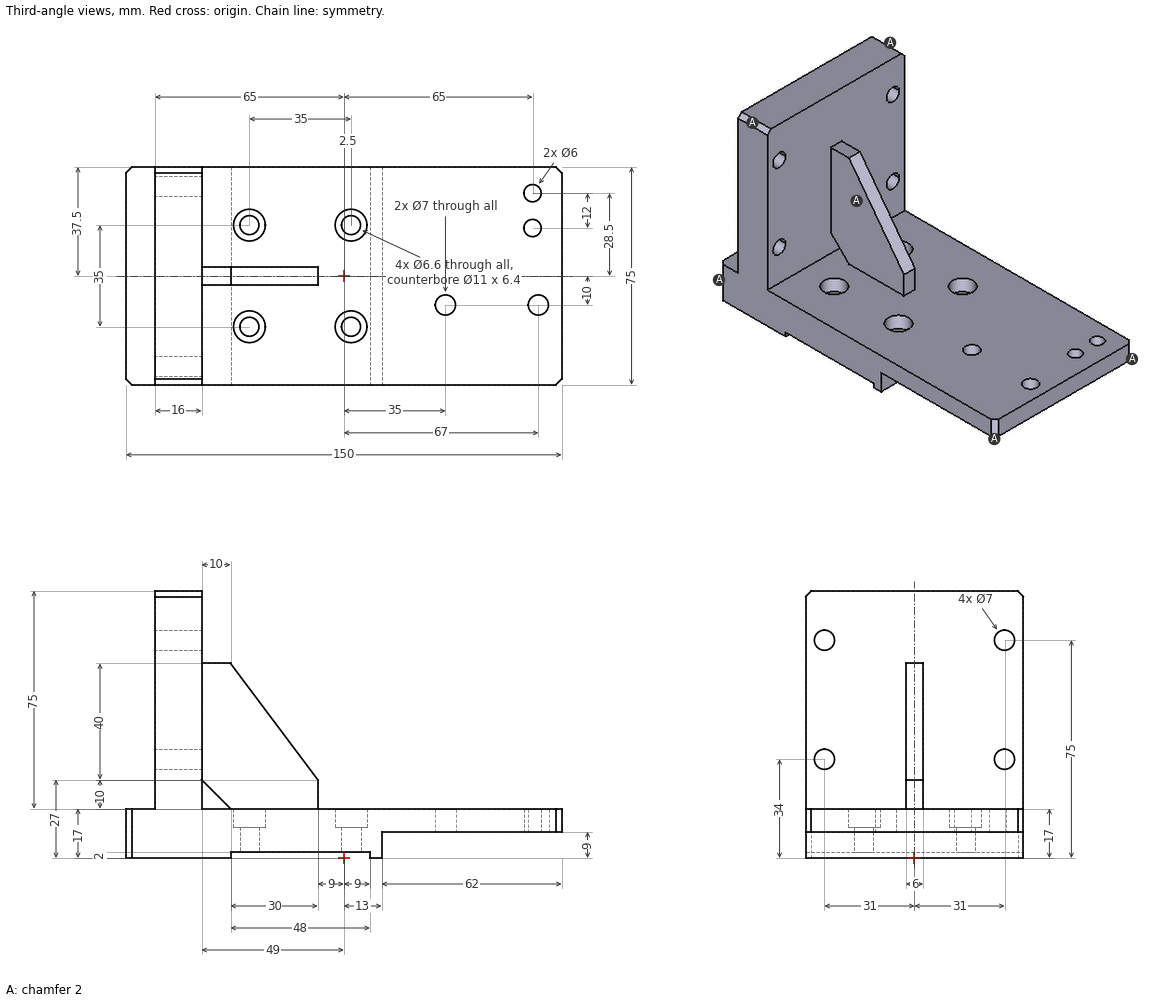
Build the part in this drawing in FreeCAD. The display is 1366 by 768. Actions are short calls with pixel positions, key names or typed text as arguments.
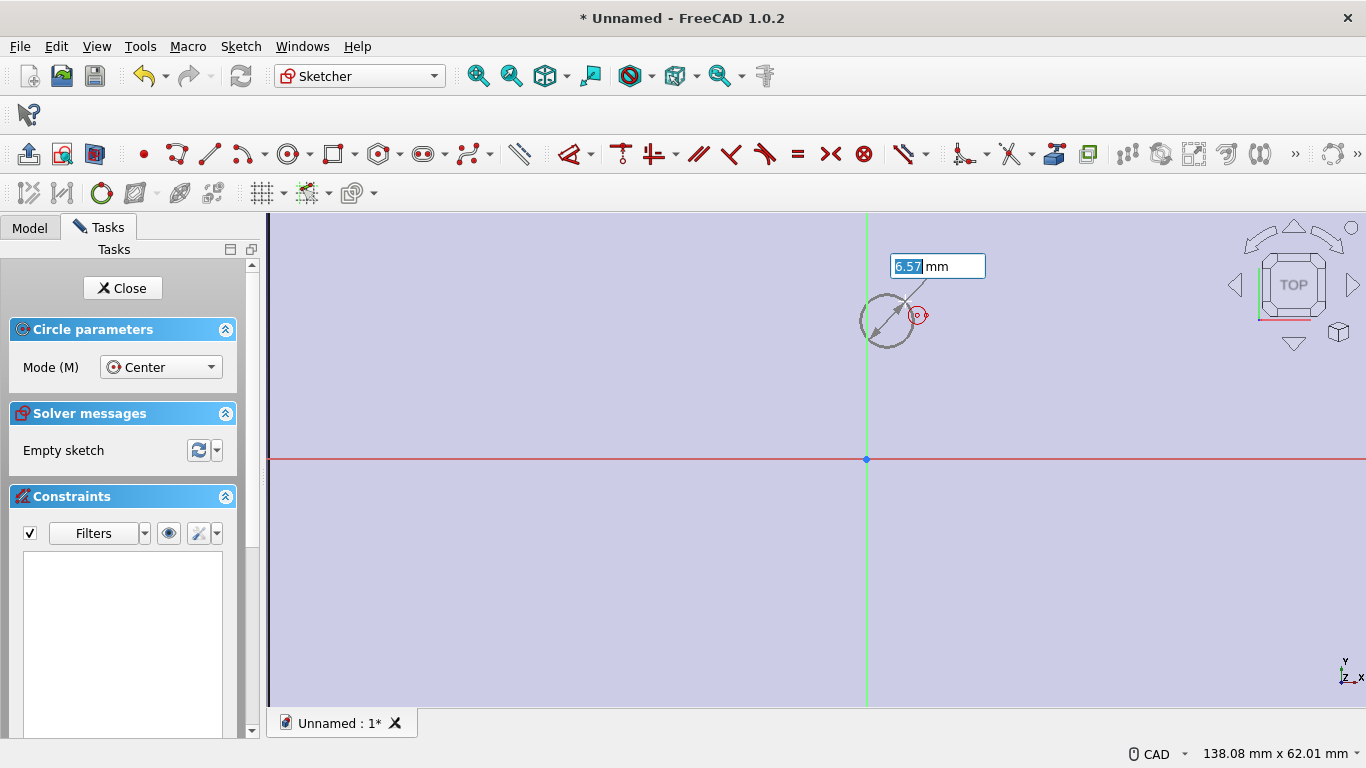
text(6.6)
key(Return)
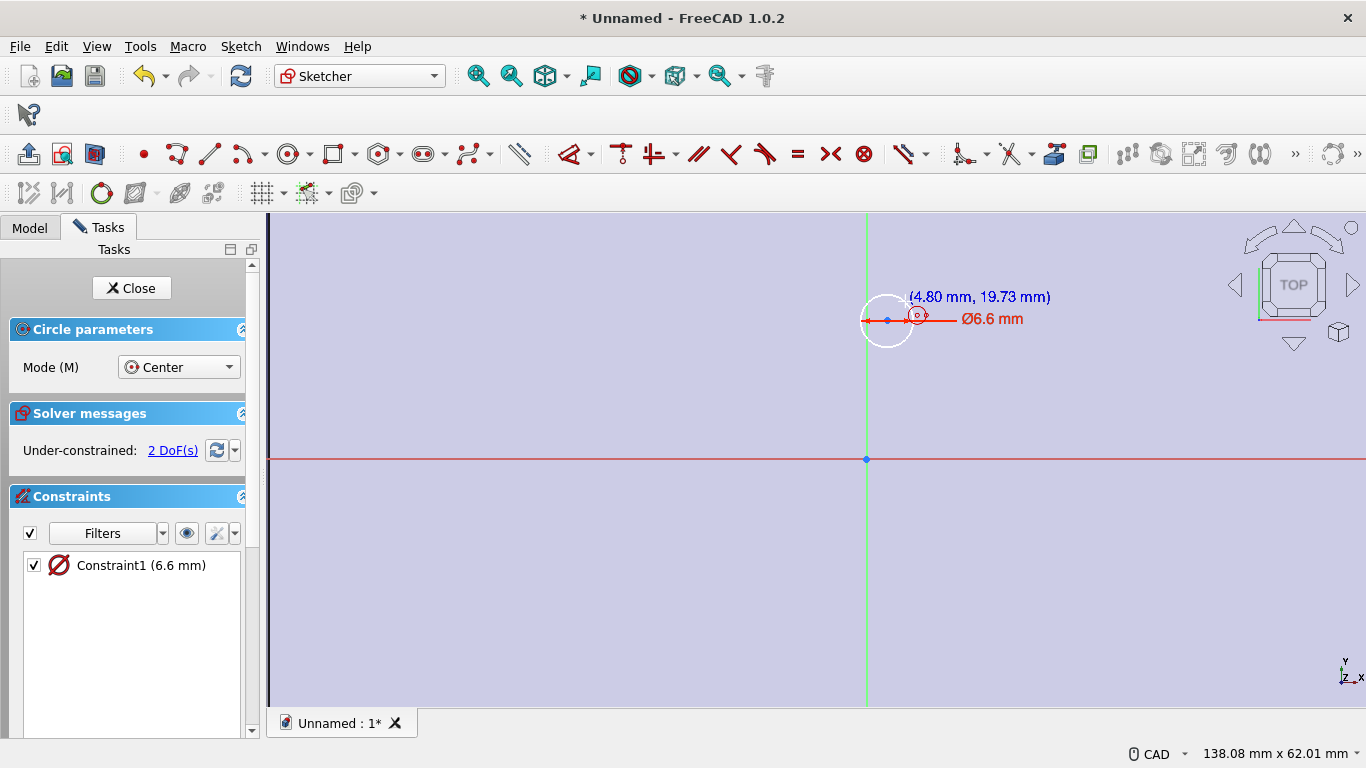
click(608, 320)
move(626, 301)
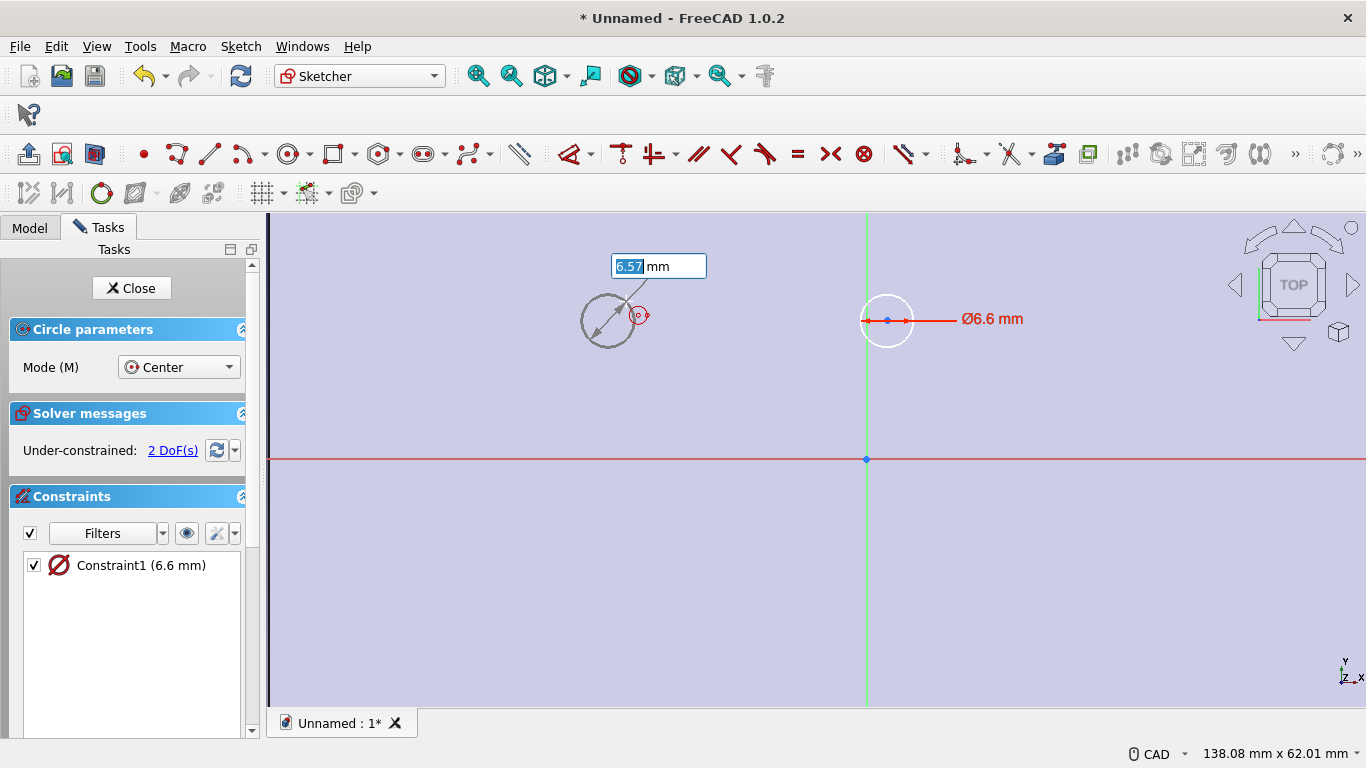
text(6.6)
key(Return)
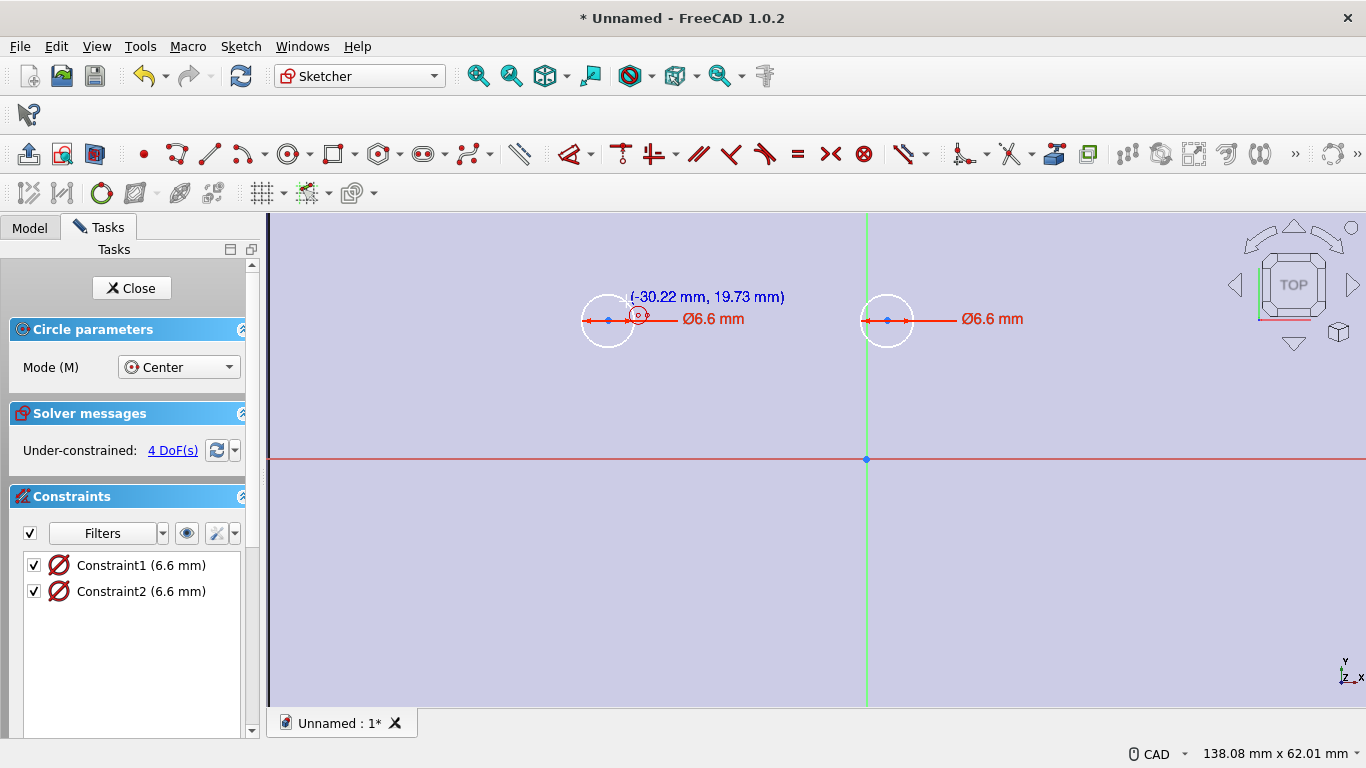
click(608, 599)
move(626, 580)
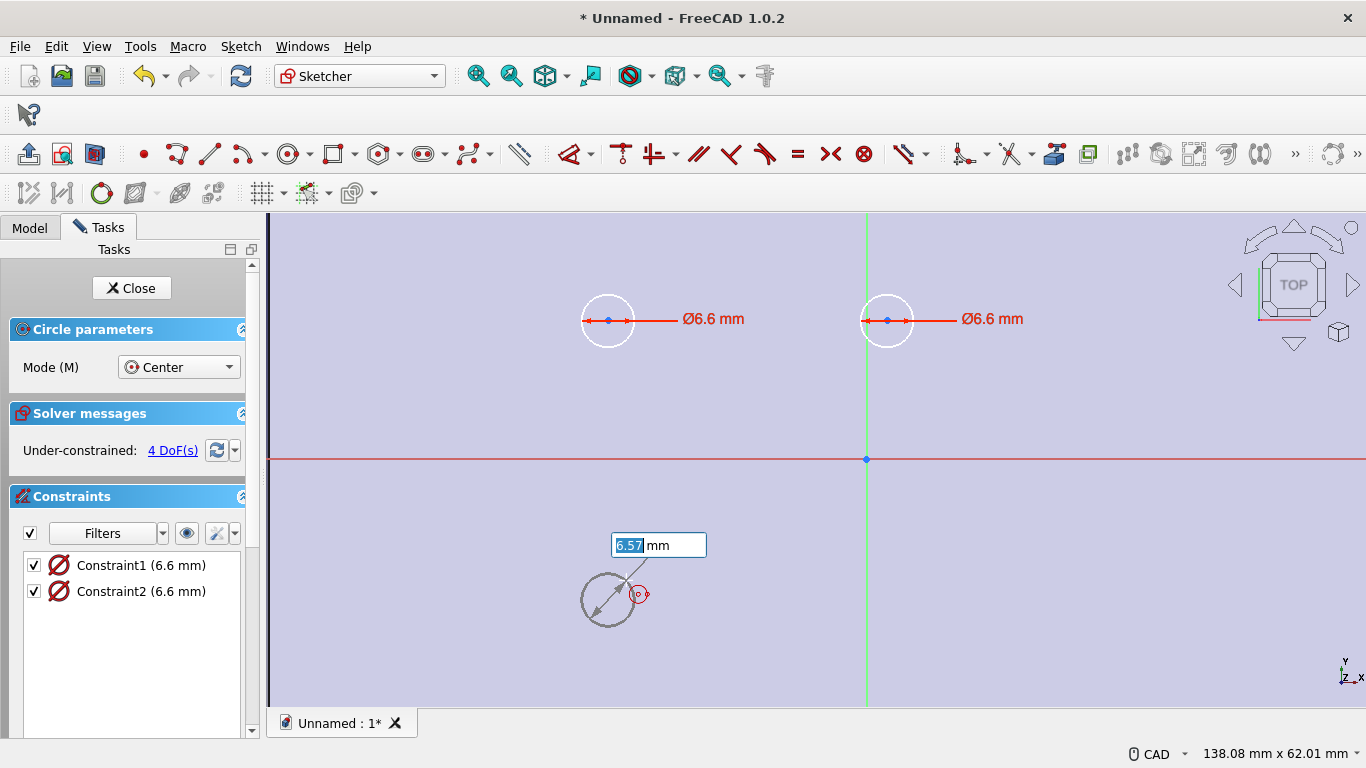
text(6.6)
key(Return)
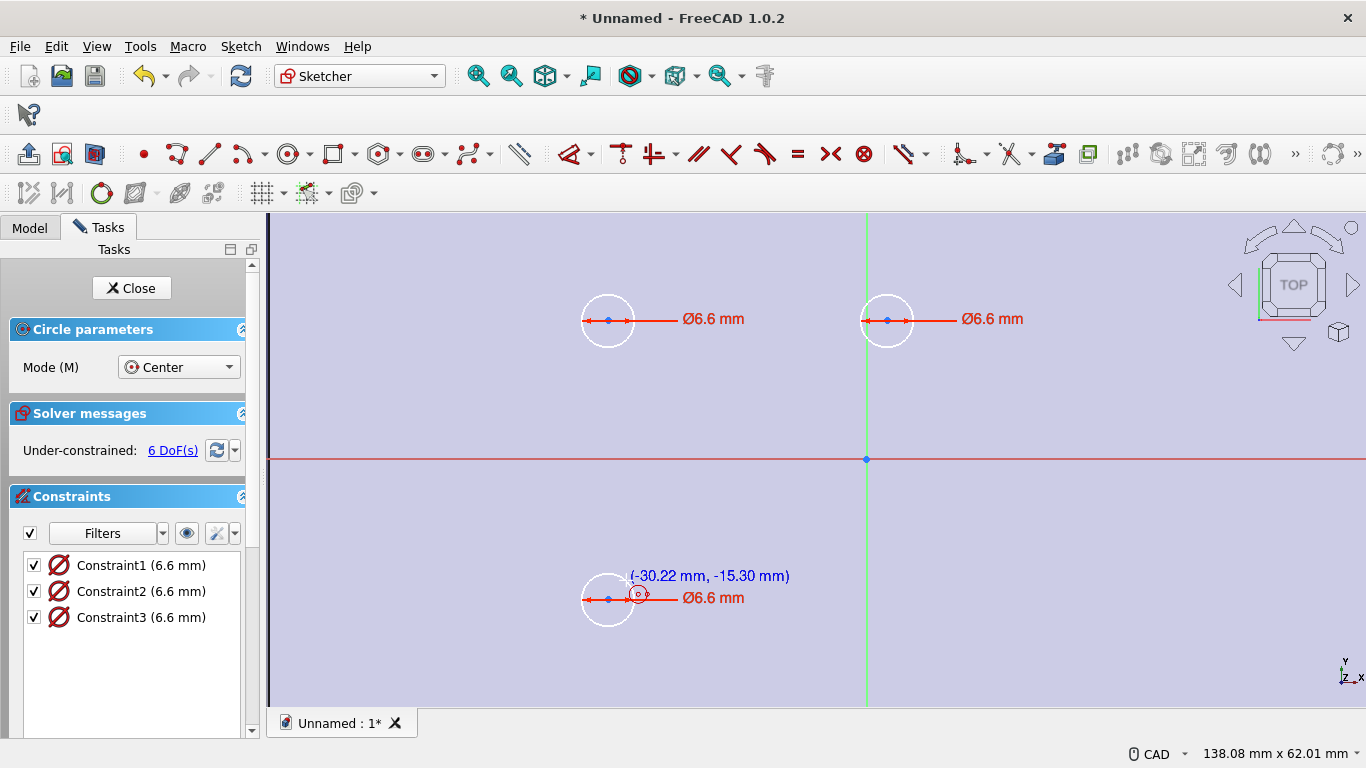
click(887, 599)
move(905, 580)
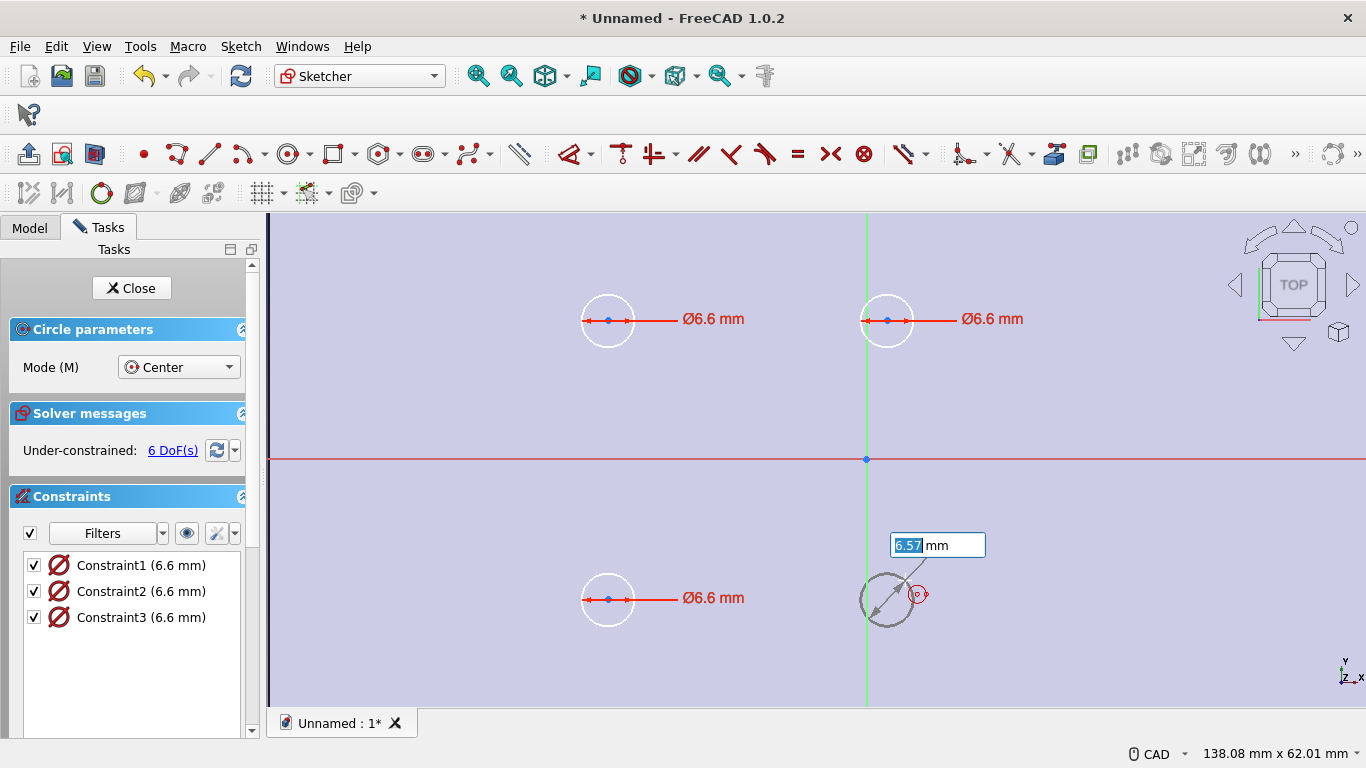
text(6.6)
key(Return)
key(Escape)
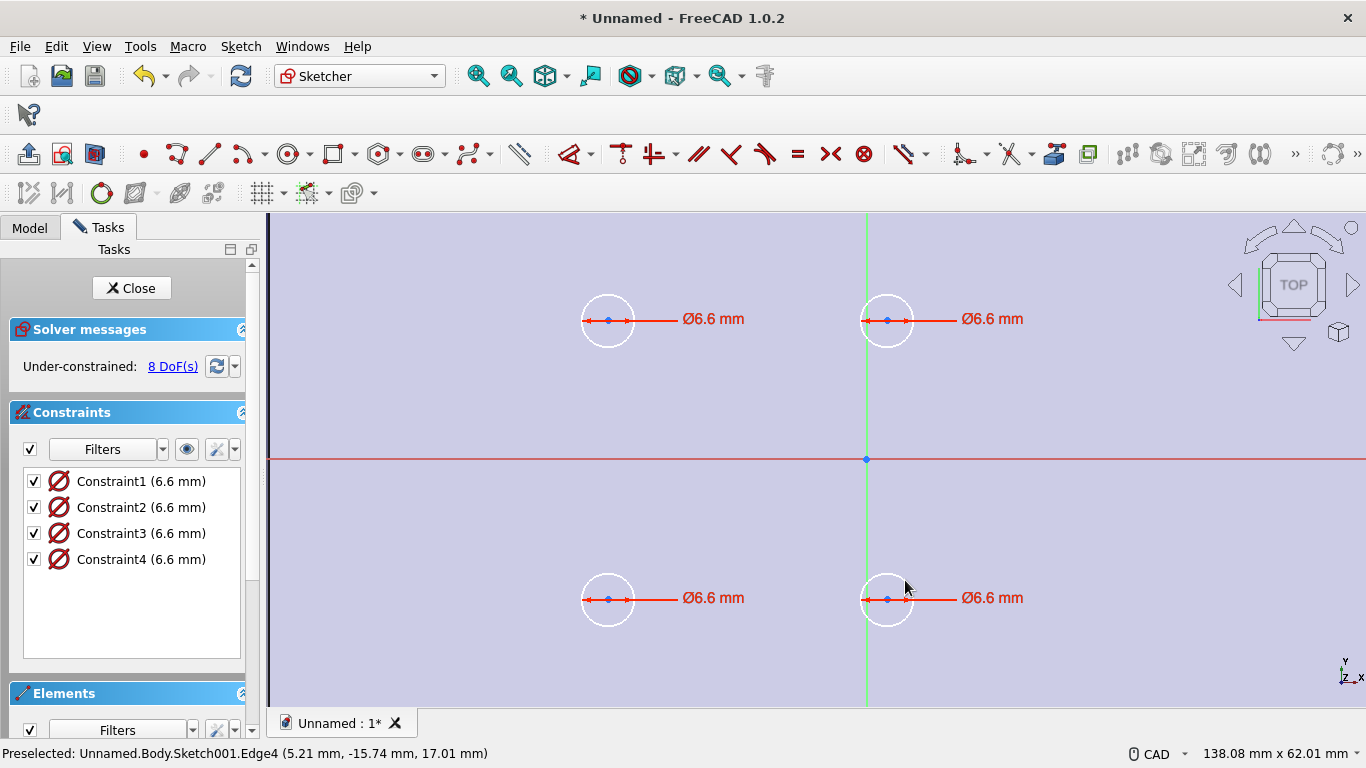
click(608, 321)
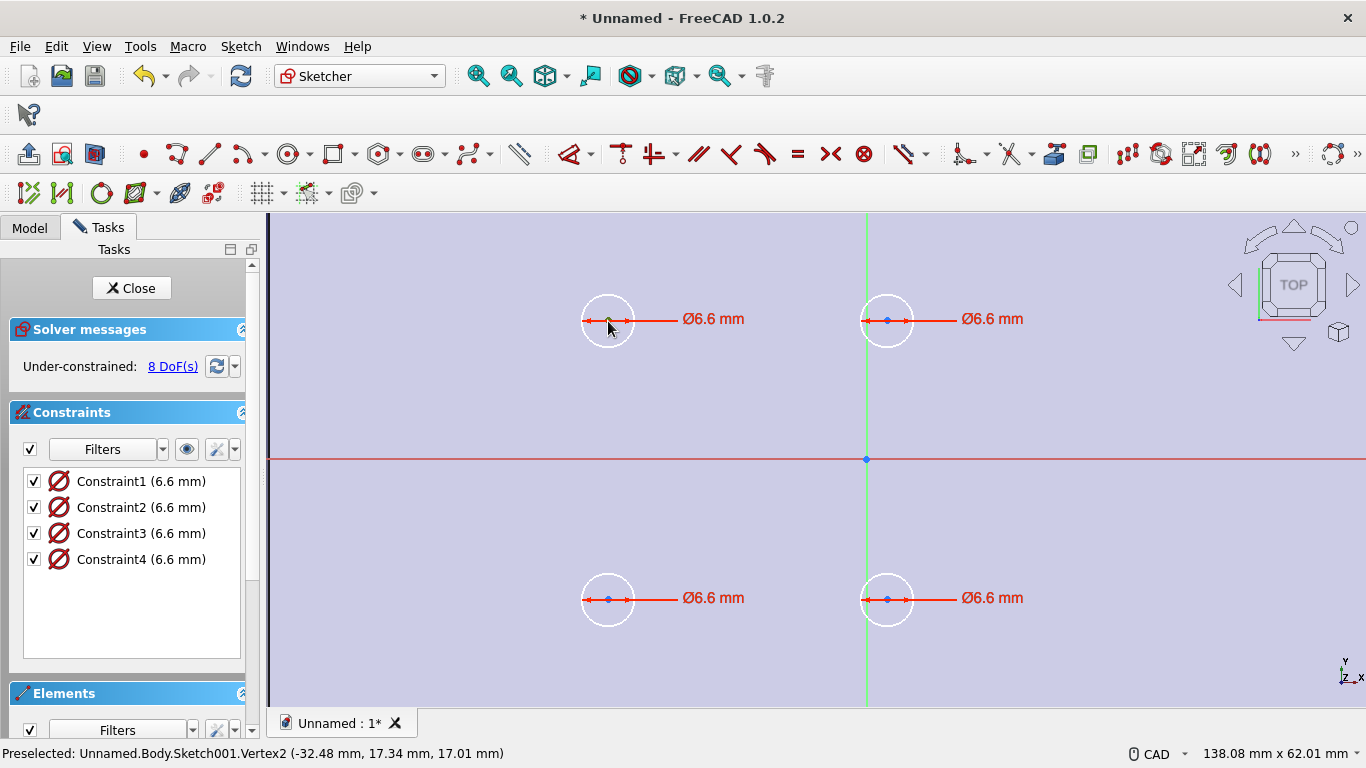
click(608, 600)